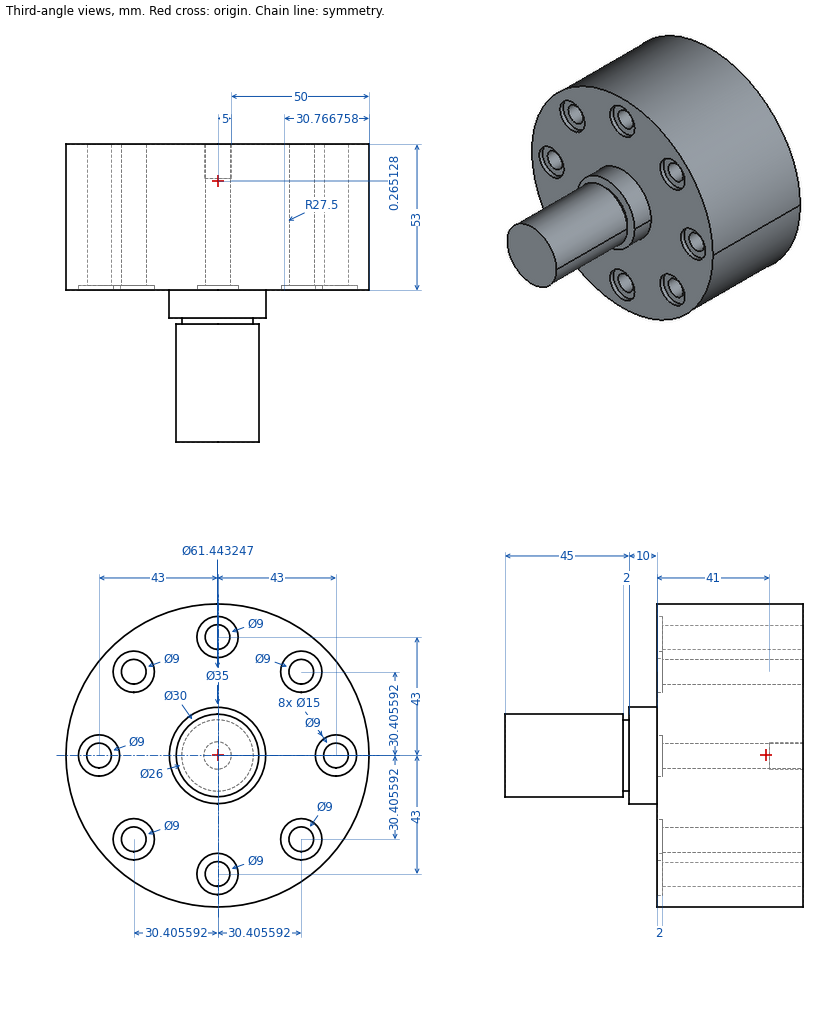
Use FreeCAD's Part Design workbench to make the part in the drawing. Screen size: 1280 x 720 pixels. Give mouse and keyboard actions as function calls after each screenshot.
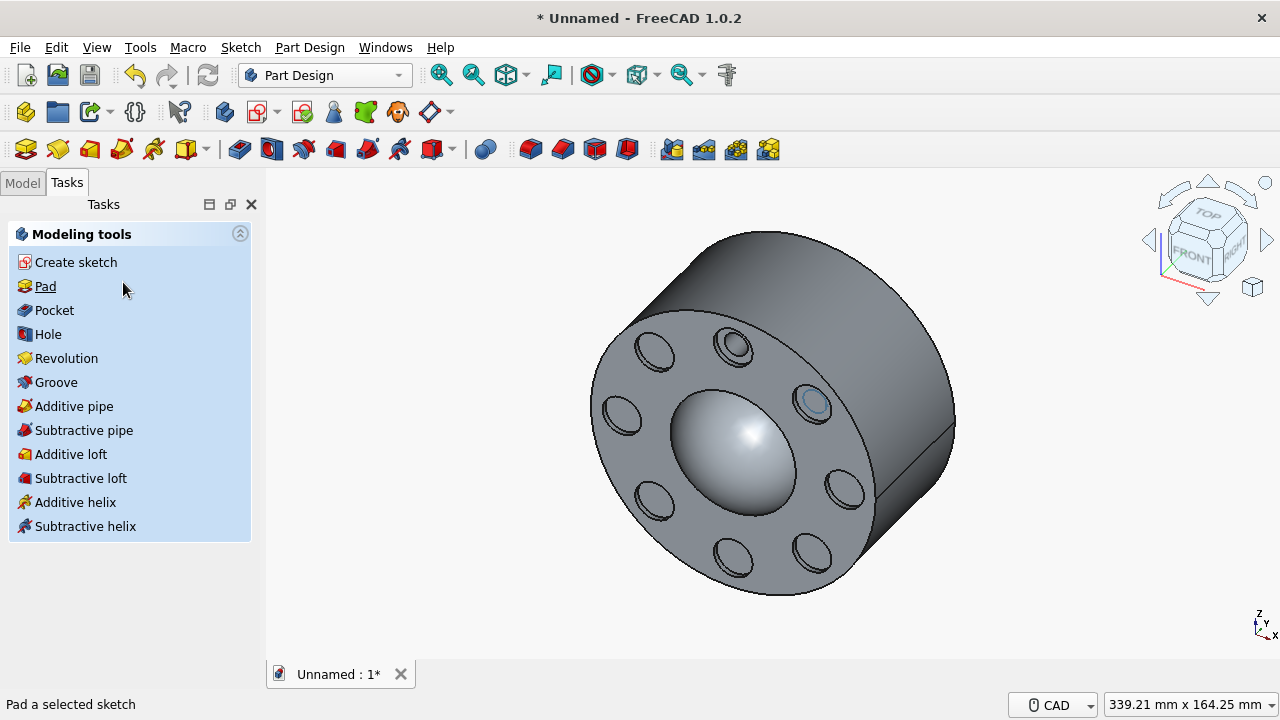
click(240, 150)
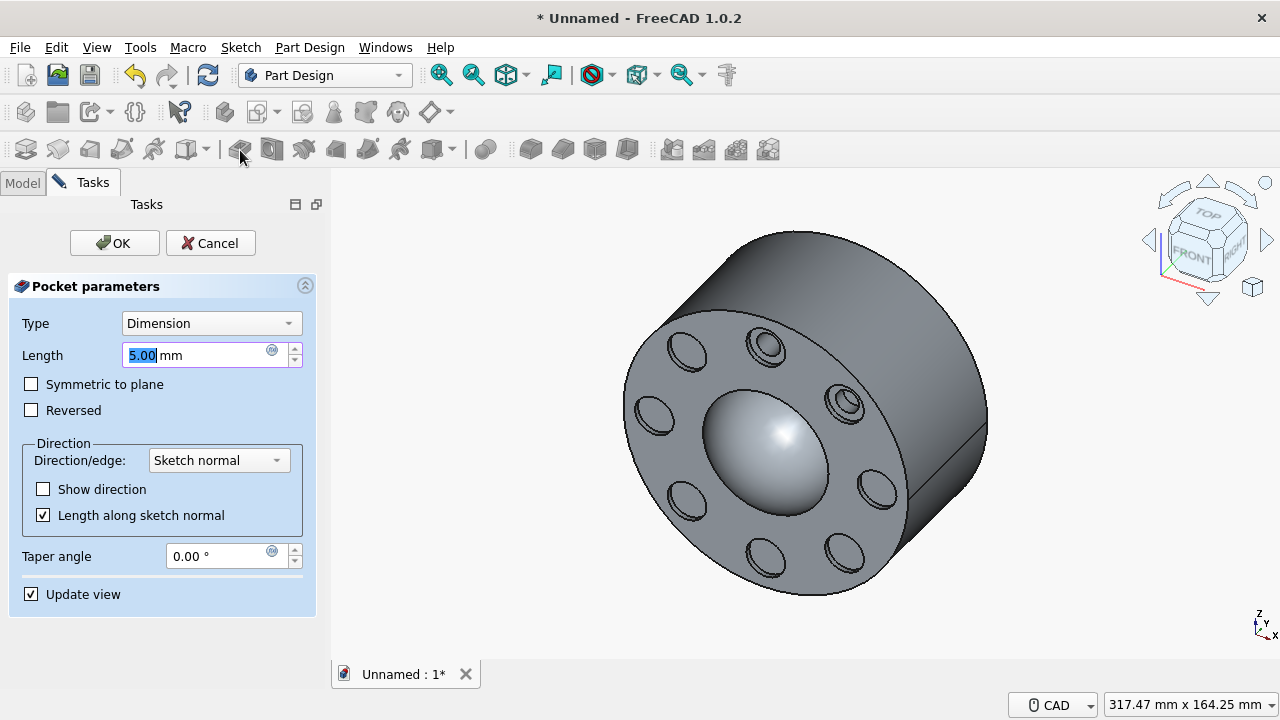
click(212, 324)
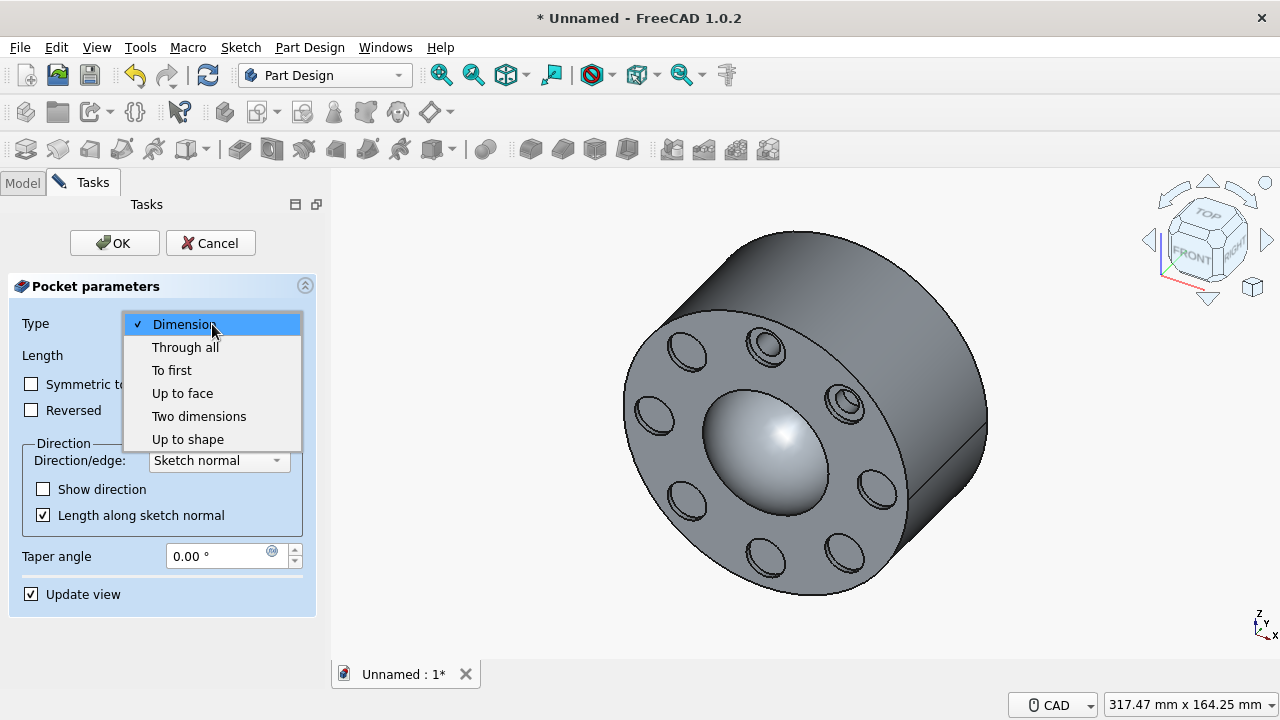
click(212, 370)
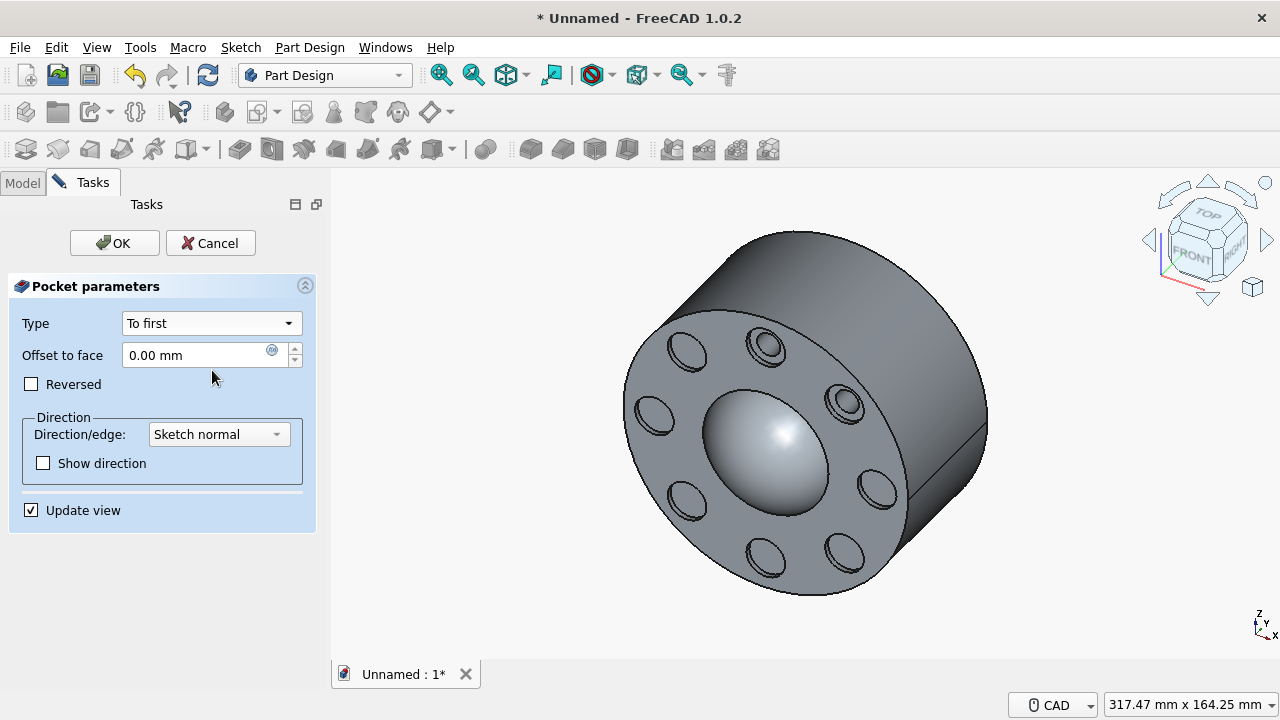
click(115, 243)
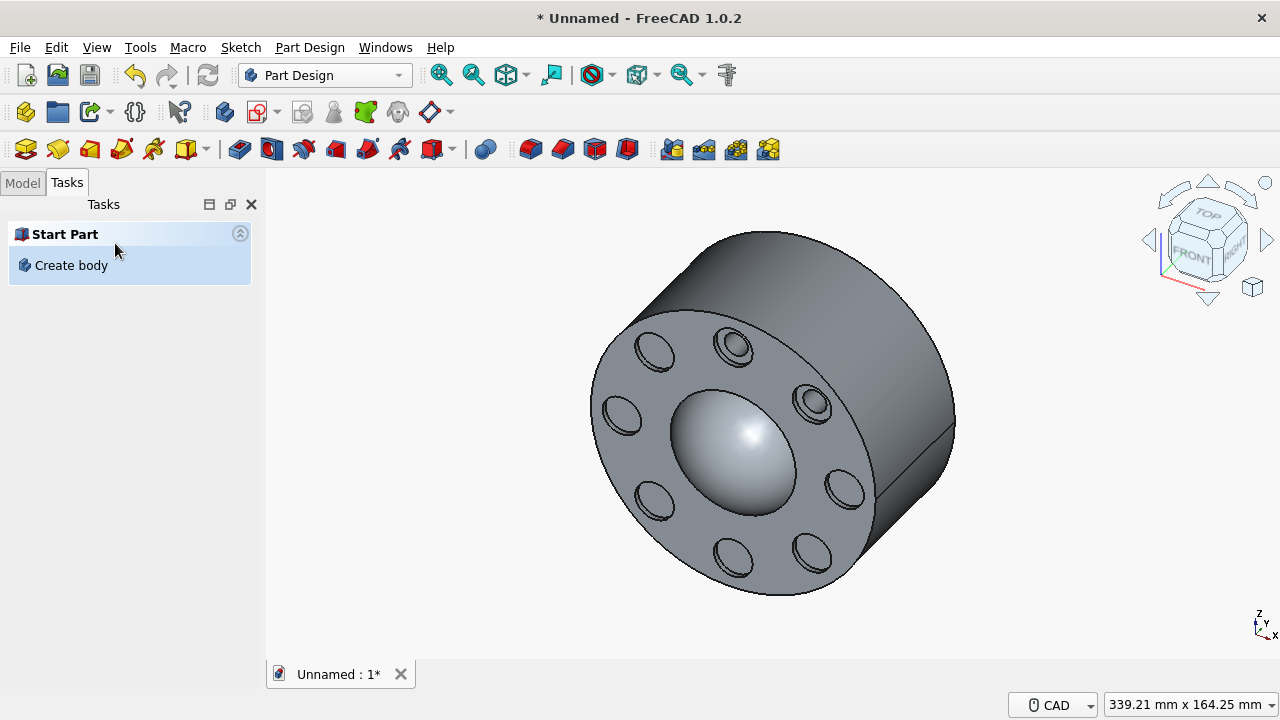
click(658, 348)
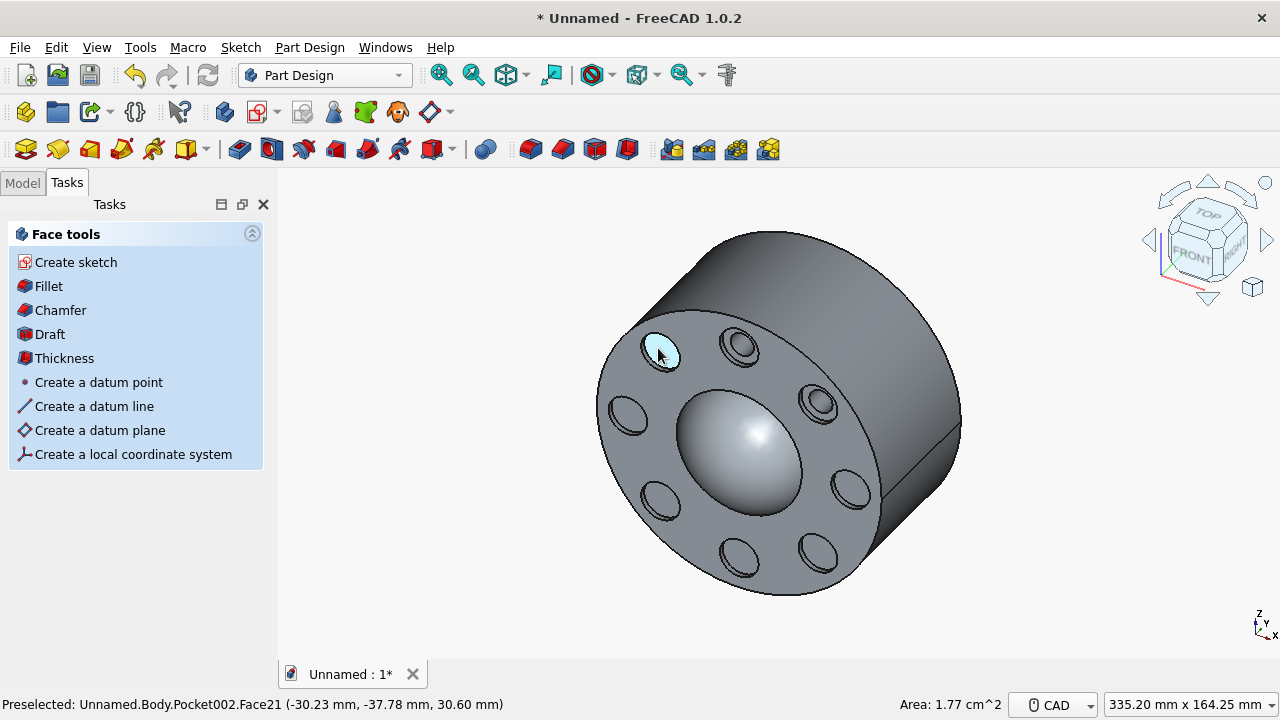
click(258, 112)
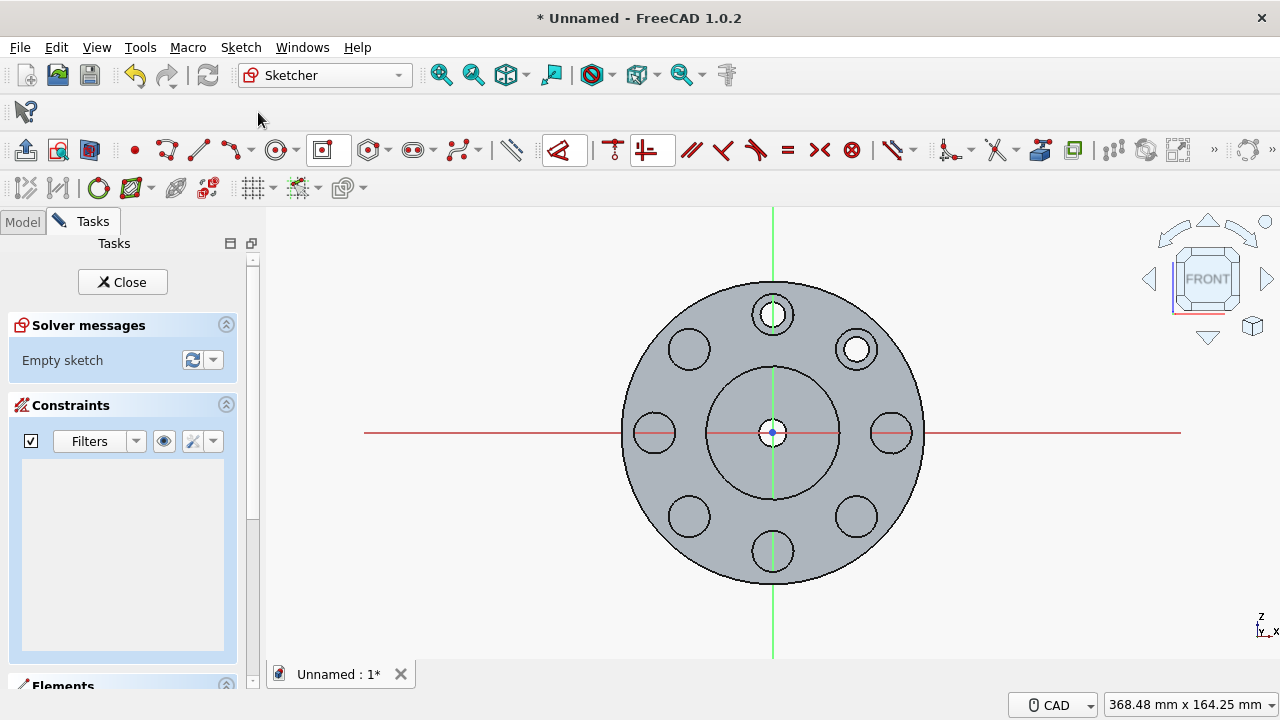
scroll(910, 433, up, 12)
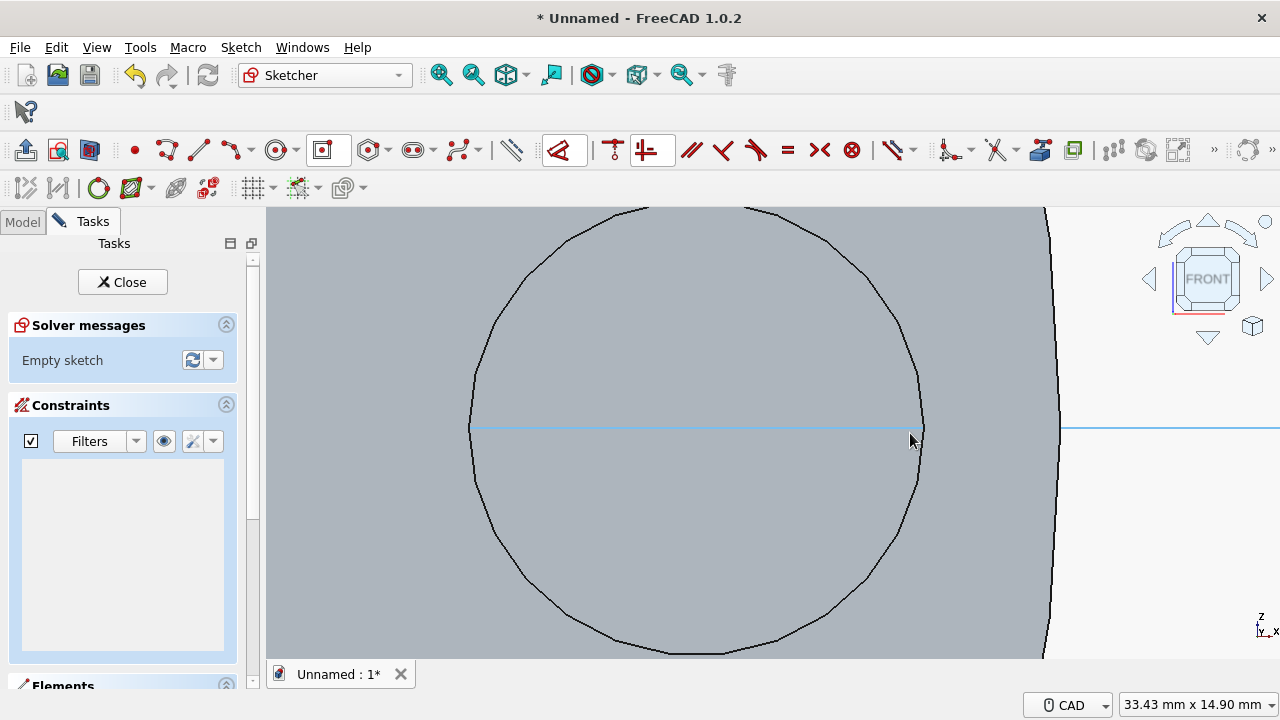
click(276, 150)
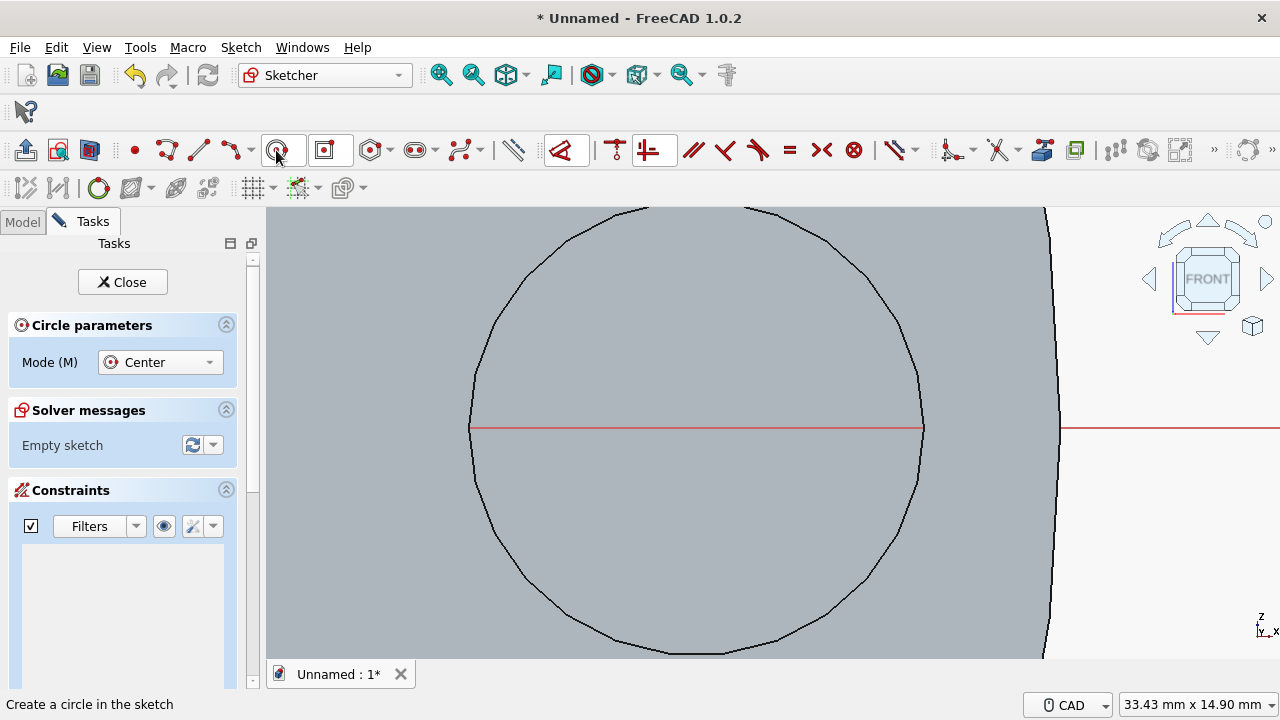
click(696, 428)
move(793, 331)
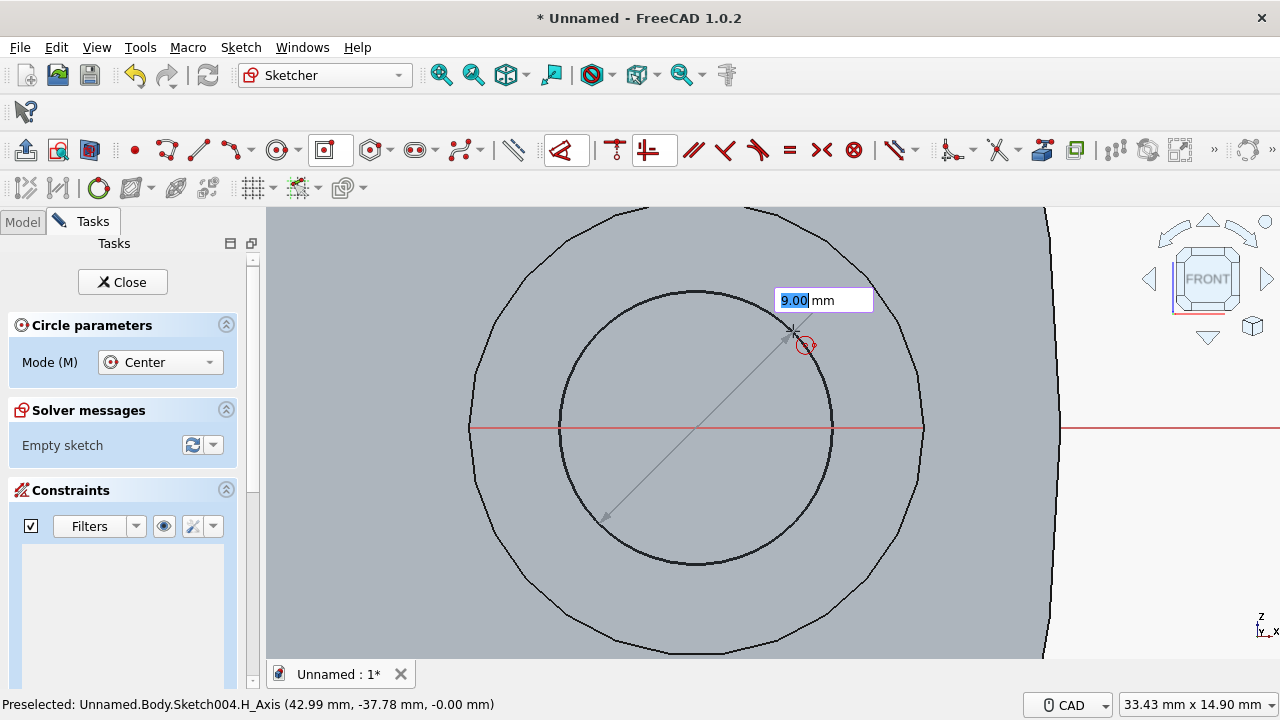
text(9)
key(Return)
key(Escape)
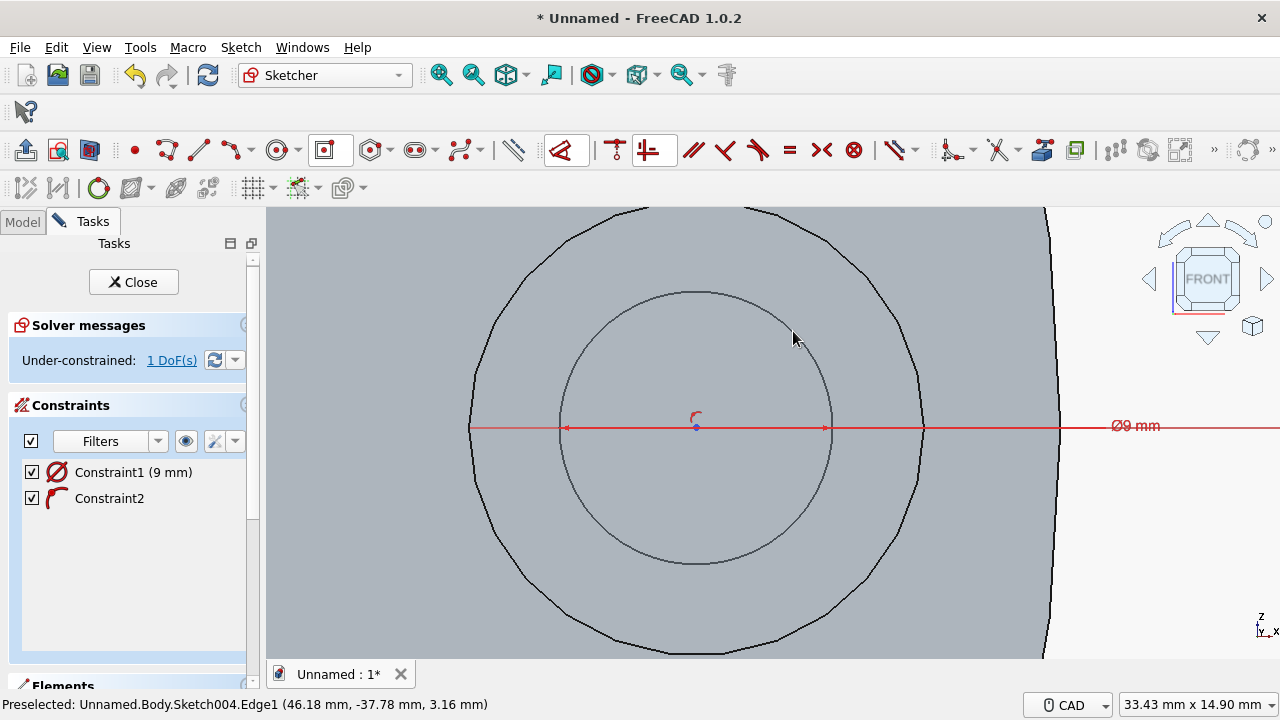
click(696, 428)